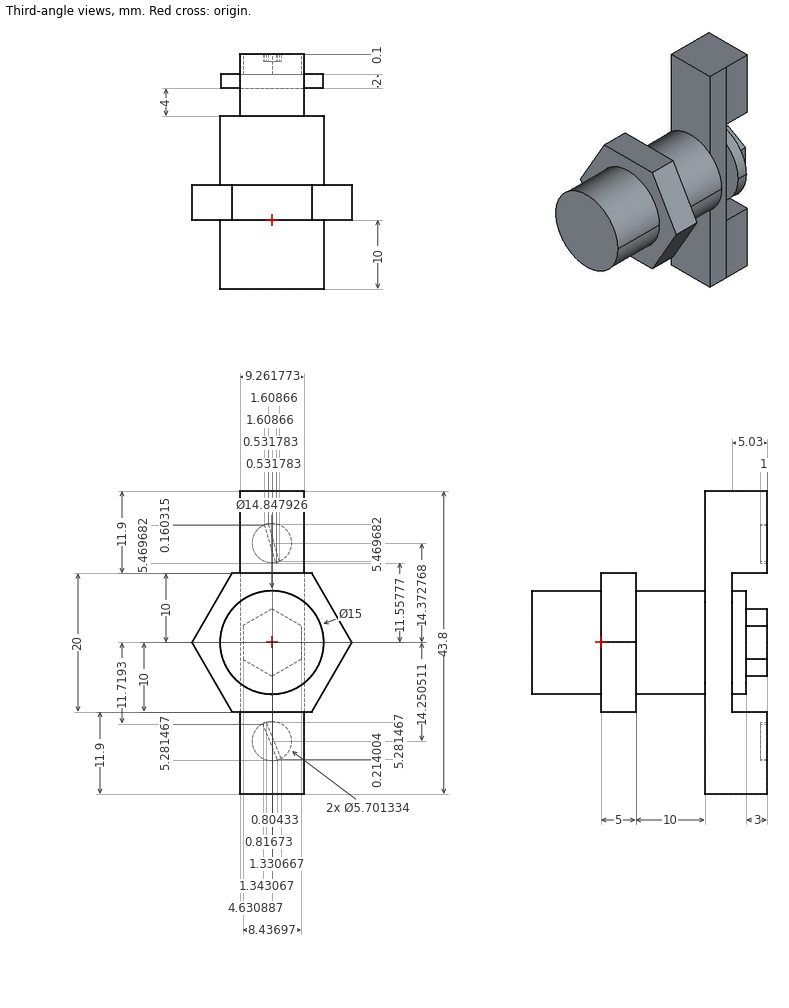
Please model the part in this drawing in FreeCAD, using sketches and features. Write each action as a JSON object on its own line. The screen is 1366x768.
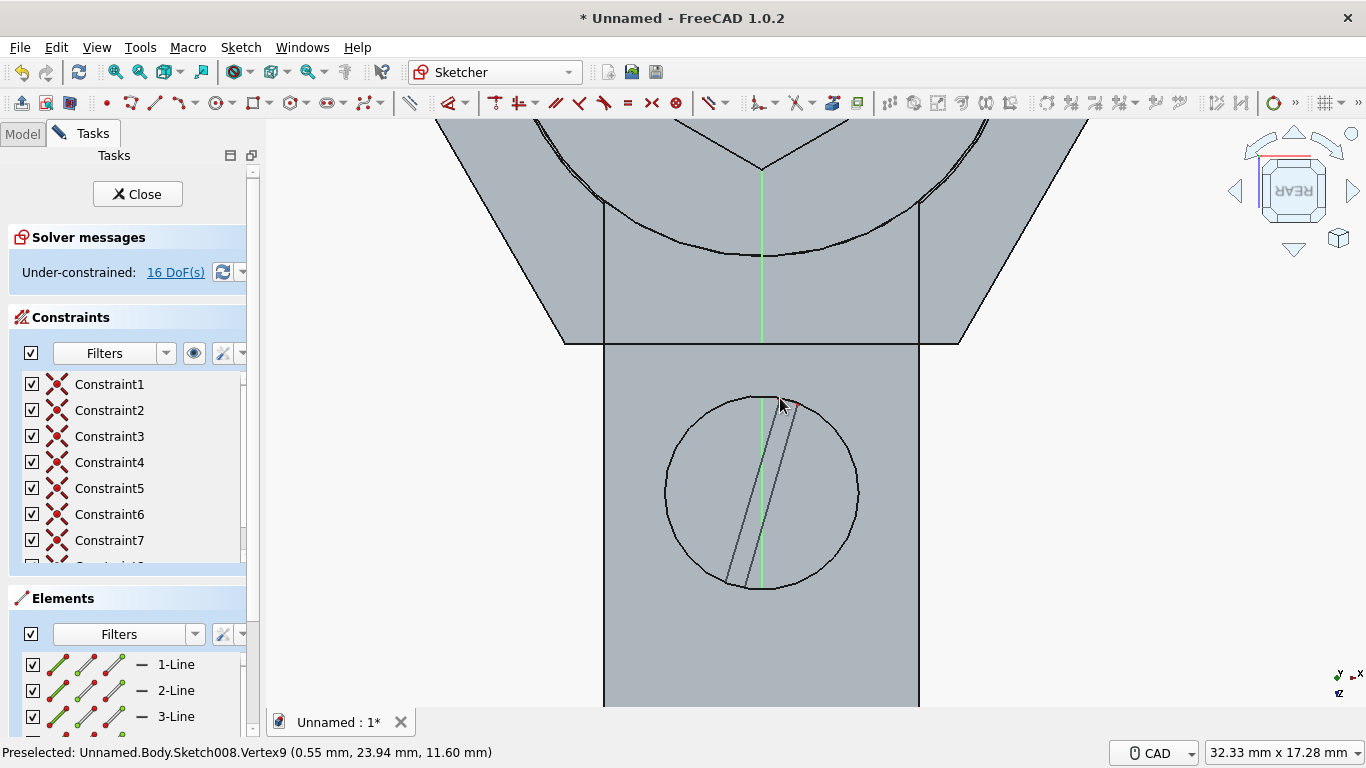
{"action": "left_click", "coordinate": [448, 104]}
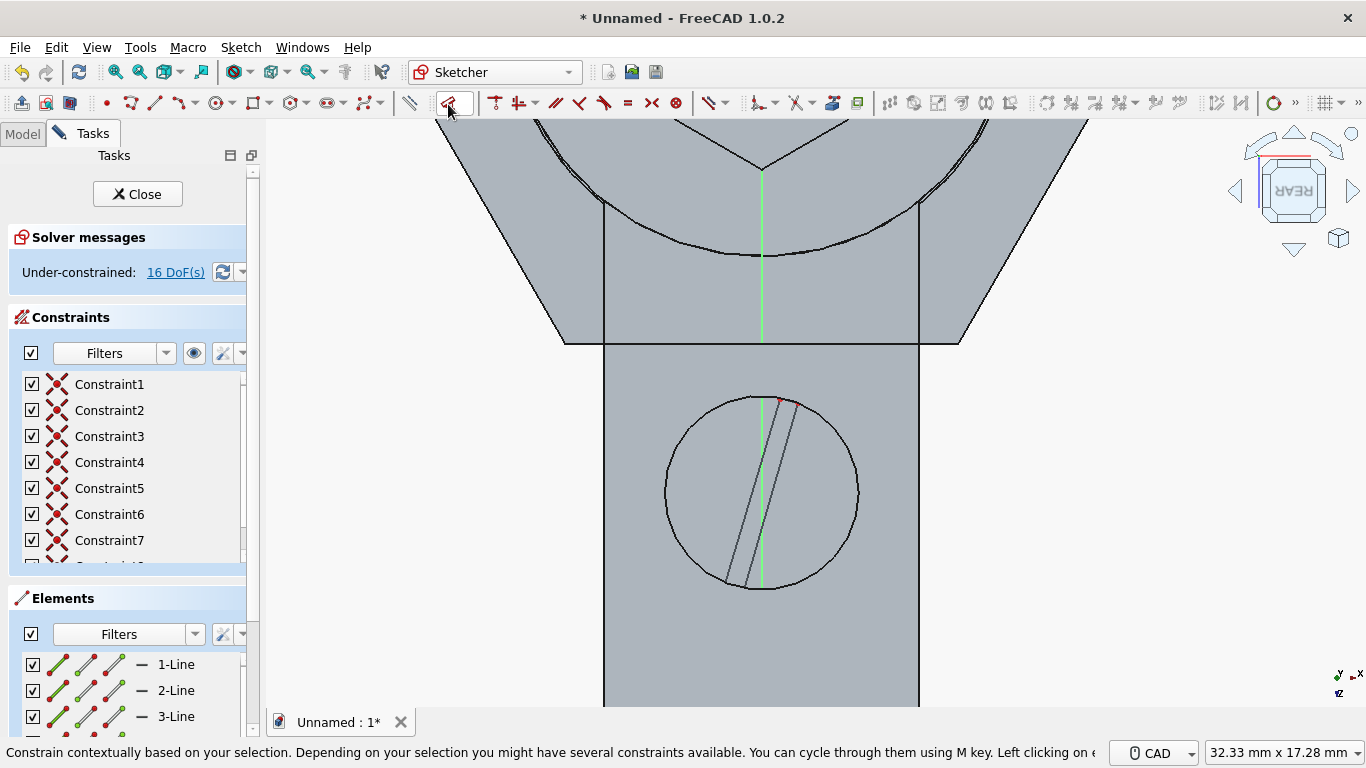
{"action": "scroll", "coordinate": [741, 588], "scroll_direction": "down", "scroll_amount": 6}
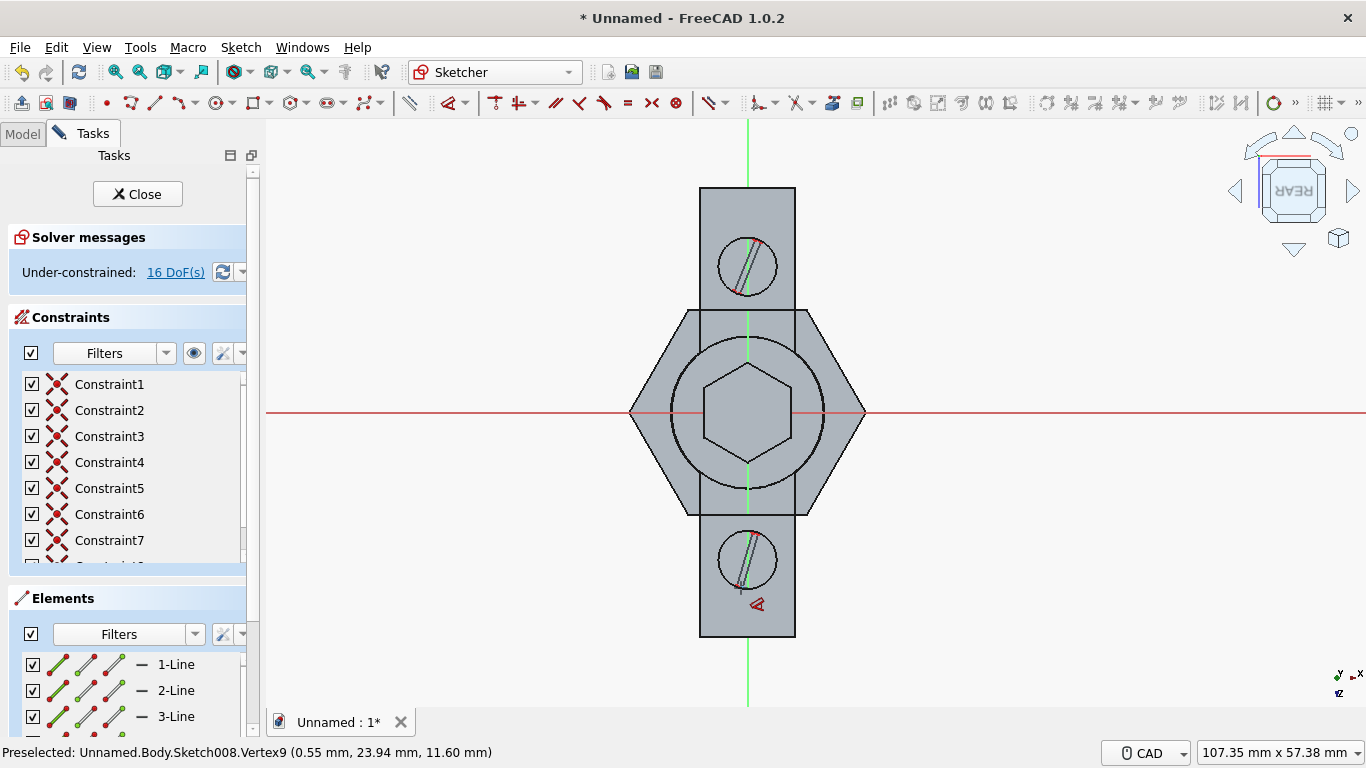
{"action": "scroll", "coordinate": [739, 295], "scroll_direction": "up", "scroll_amount": 8}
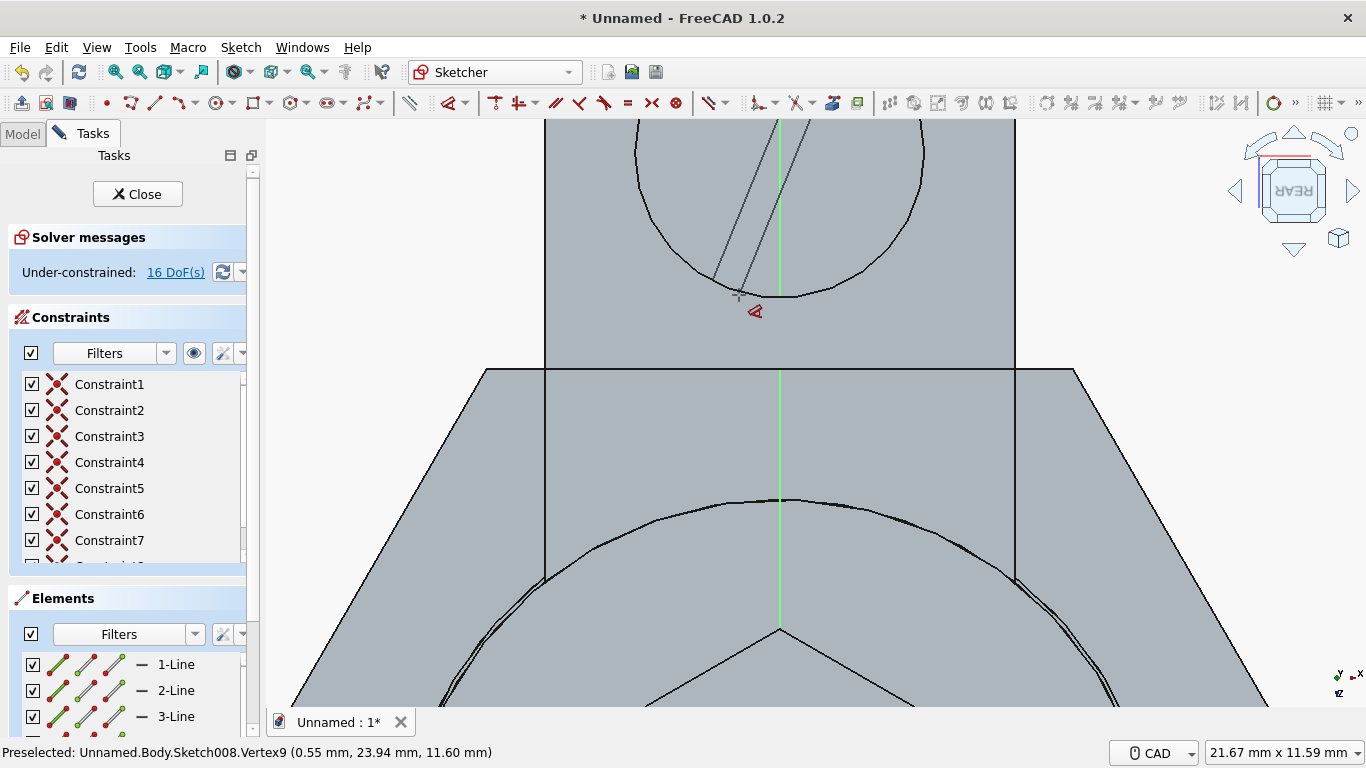
{"action": "left_click", "coordinate": [739, 295]}
{"action": "left_click", "coordinate": [745, 237]}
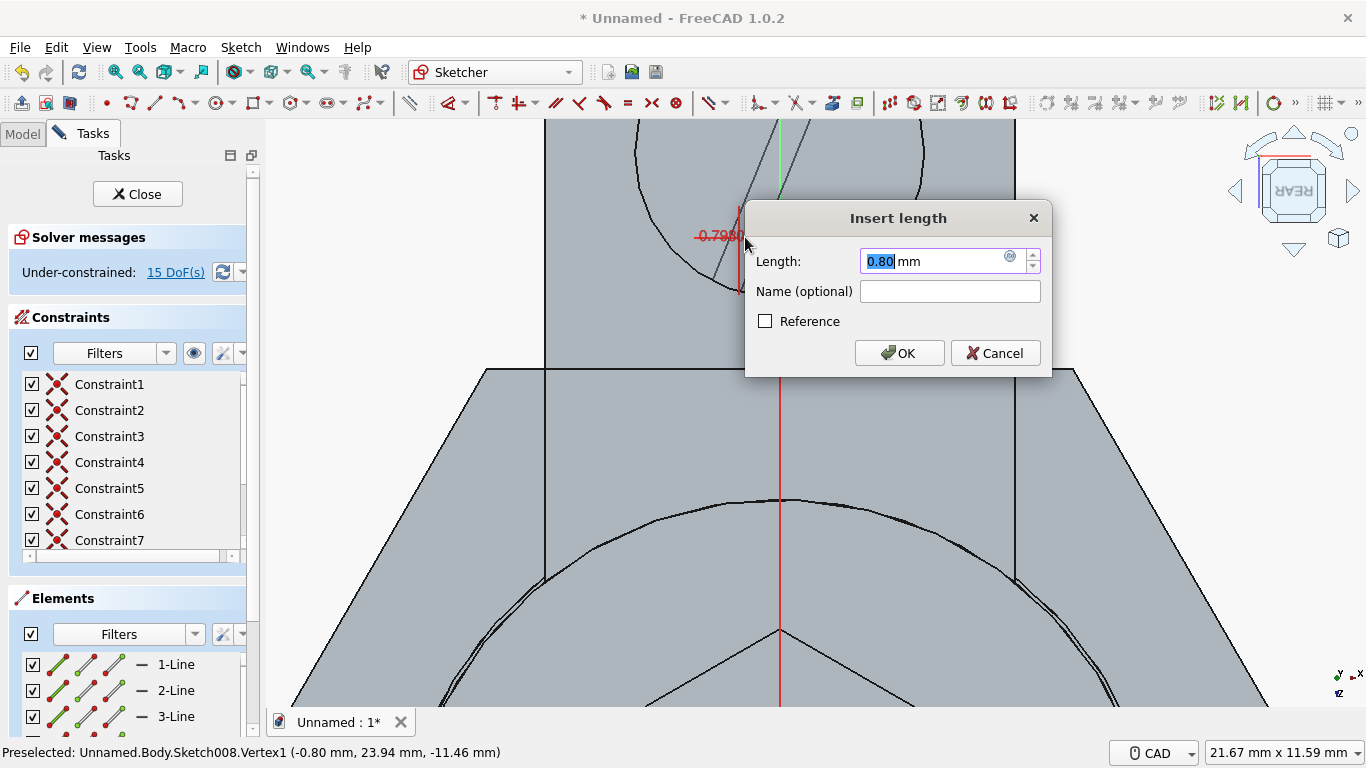
{"action": "type", "text": "0.81673"}
{"action": "key", "text": "Return"}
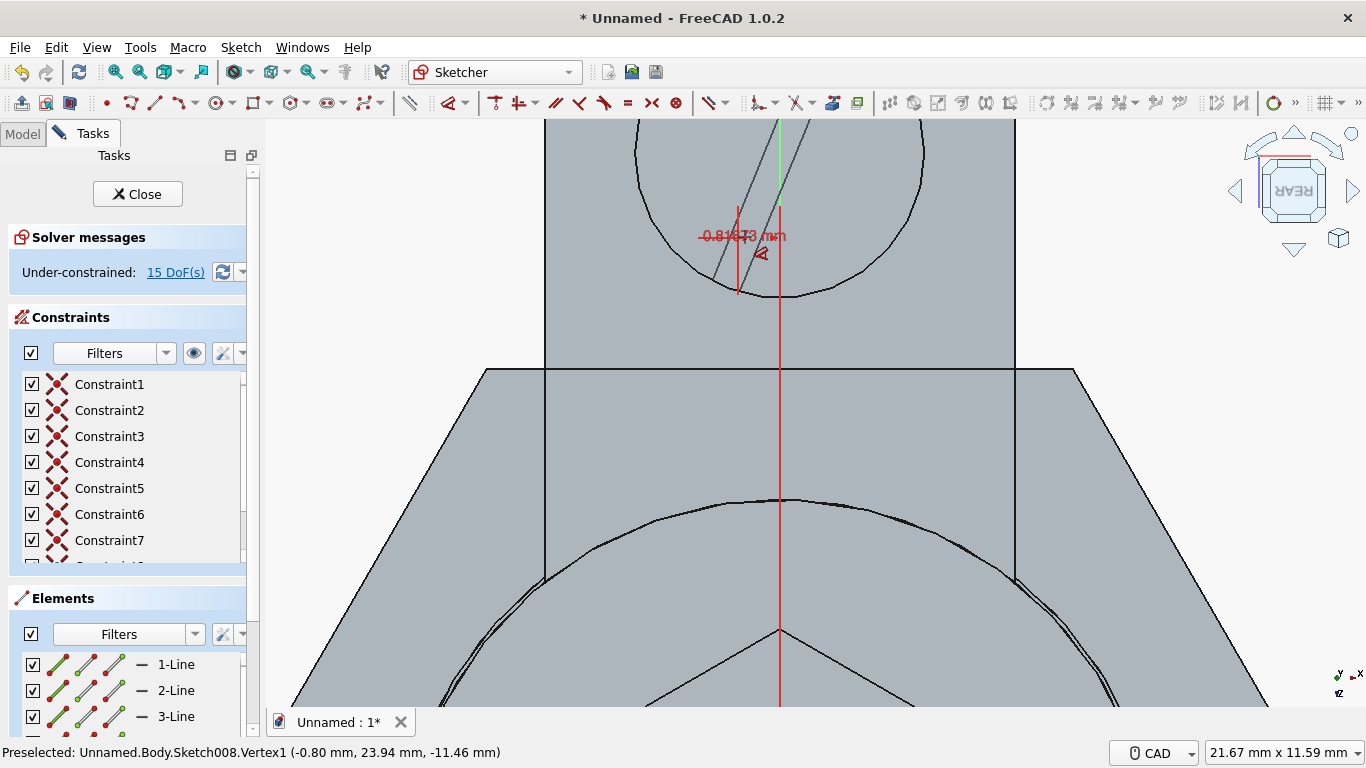
{"action": "scroll", "coordinate": [739, 295], "scroll_direction": "down", "scroll_amount": 8}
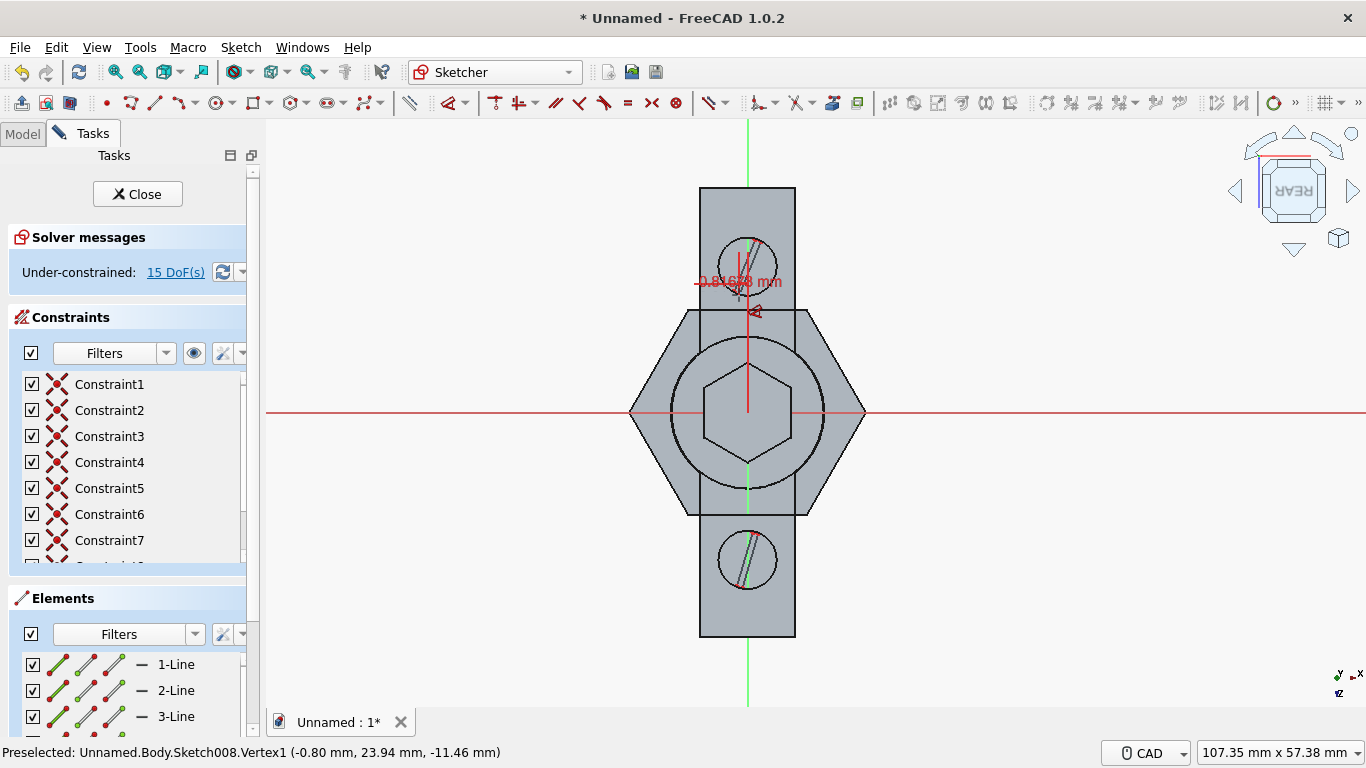
{"action": "scroll", "coordinate": [756, 239], "scroll_direction": "up", "scroll_amount": 8}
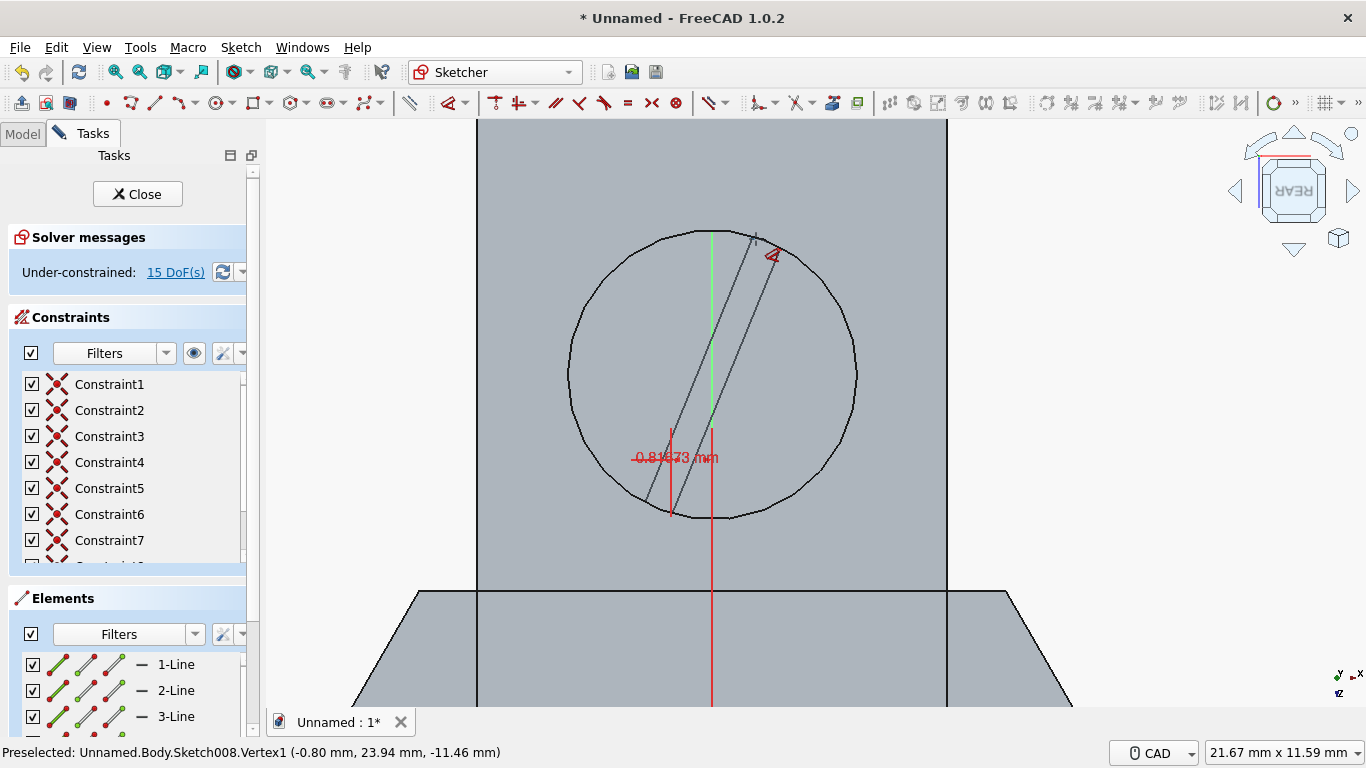
{"action": "left_click", "coordinate": [753, 236]}
{"action": "left_click", "coordinate": [733, 202]}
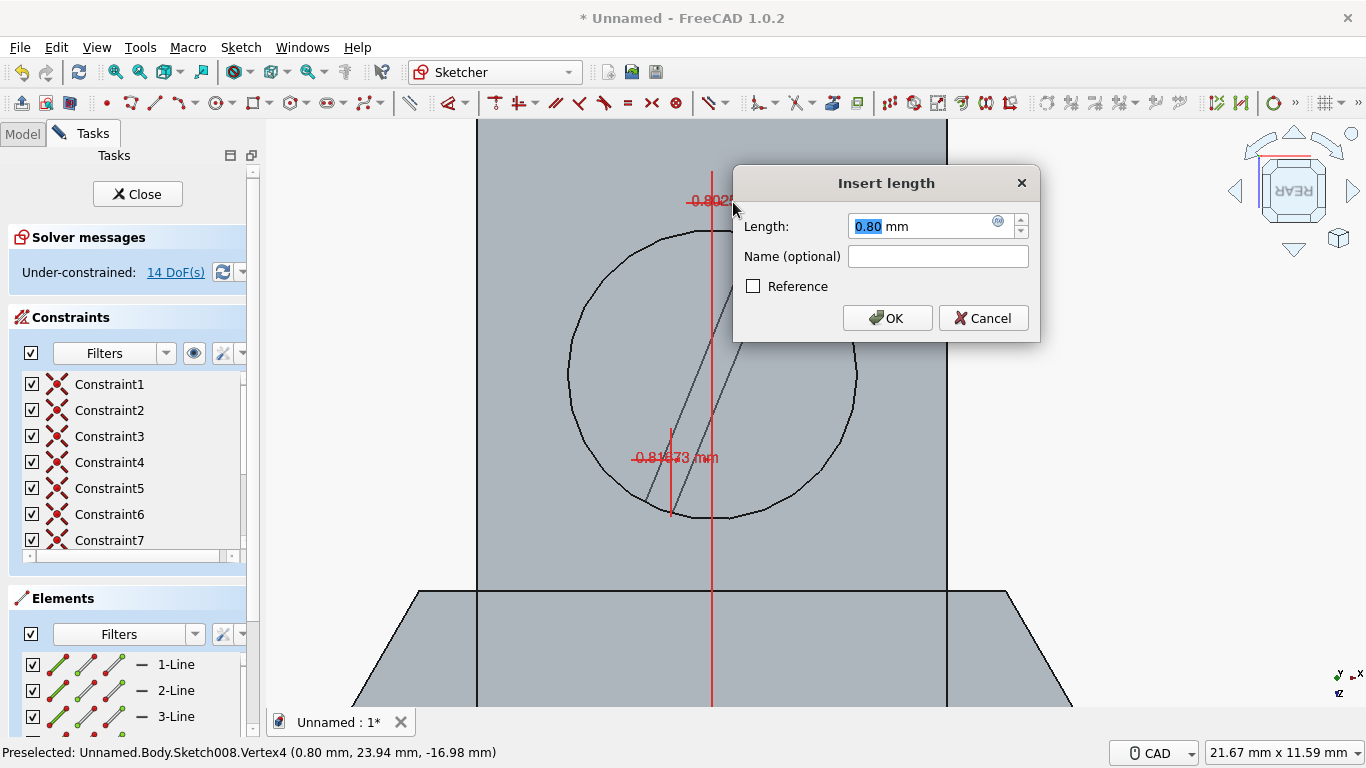
{"action": "type", "text": "0.80433"}
{"action": "key", "text": "Return"}